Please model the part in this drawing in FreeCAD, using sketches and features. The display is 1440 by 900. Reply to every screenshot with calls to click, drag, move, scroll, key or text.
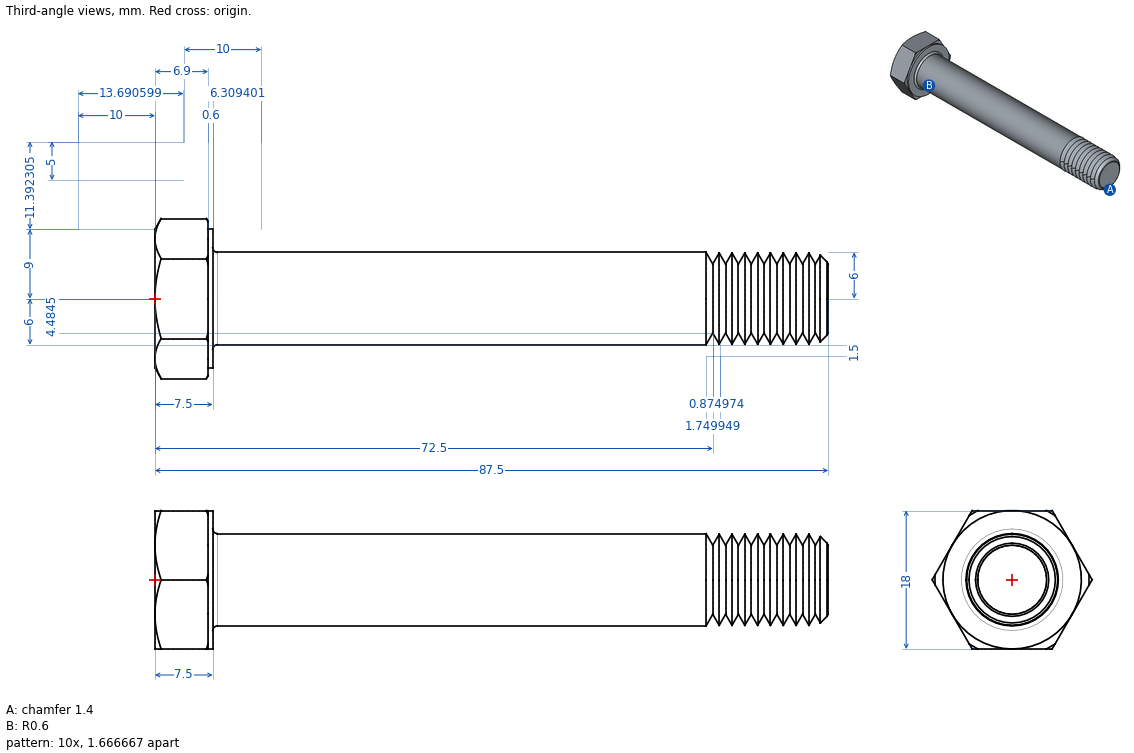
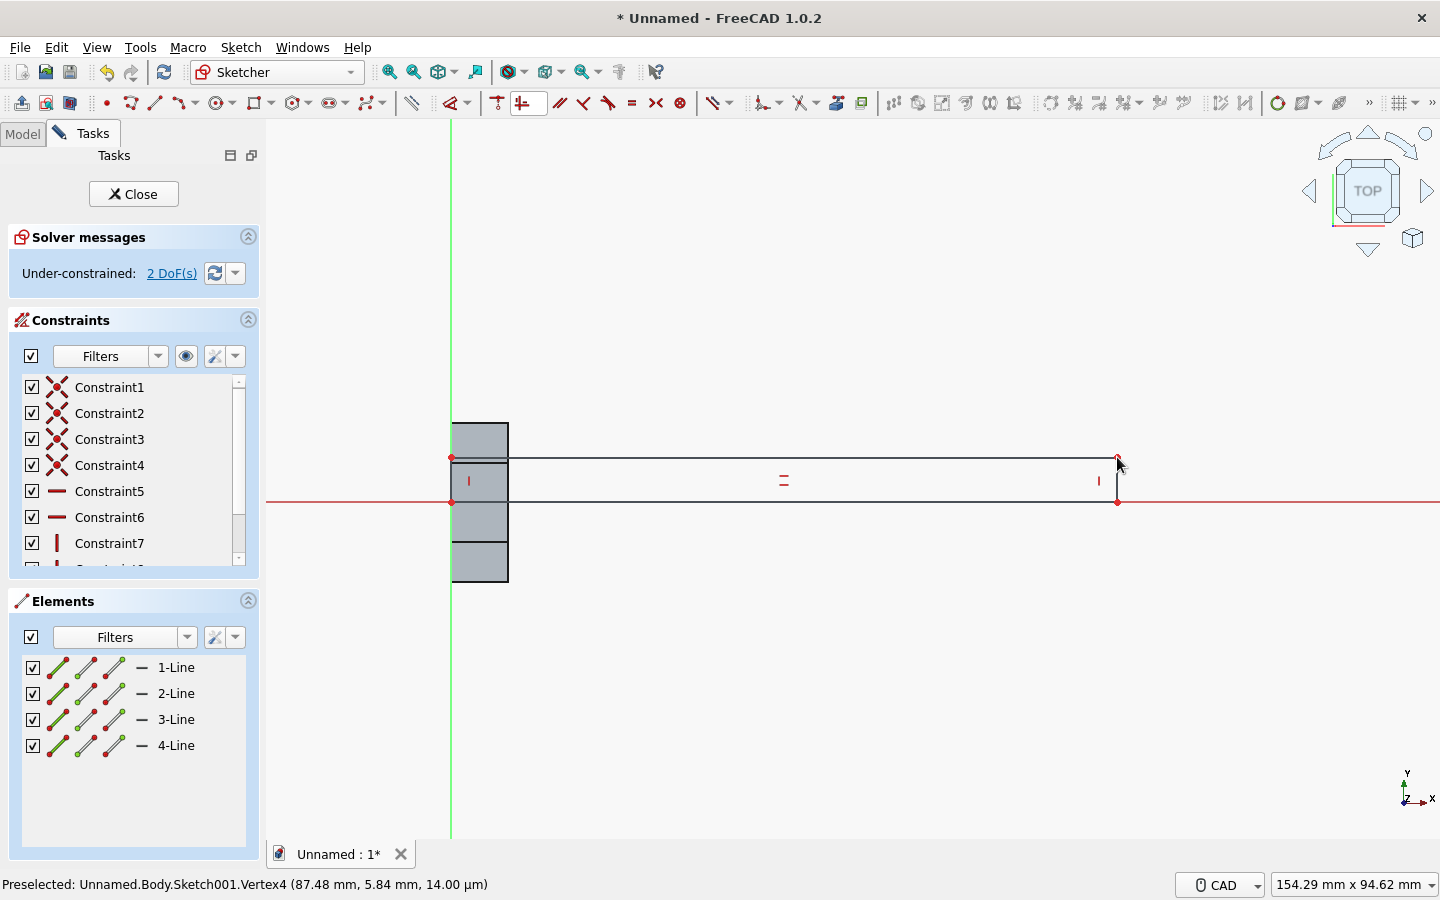
click(450, 104)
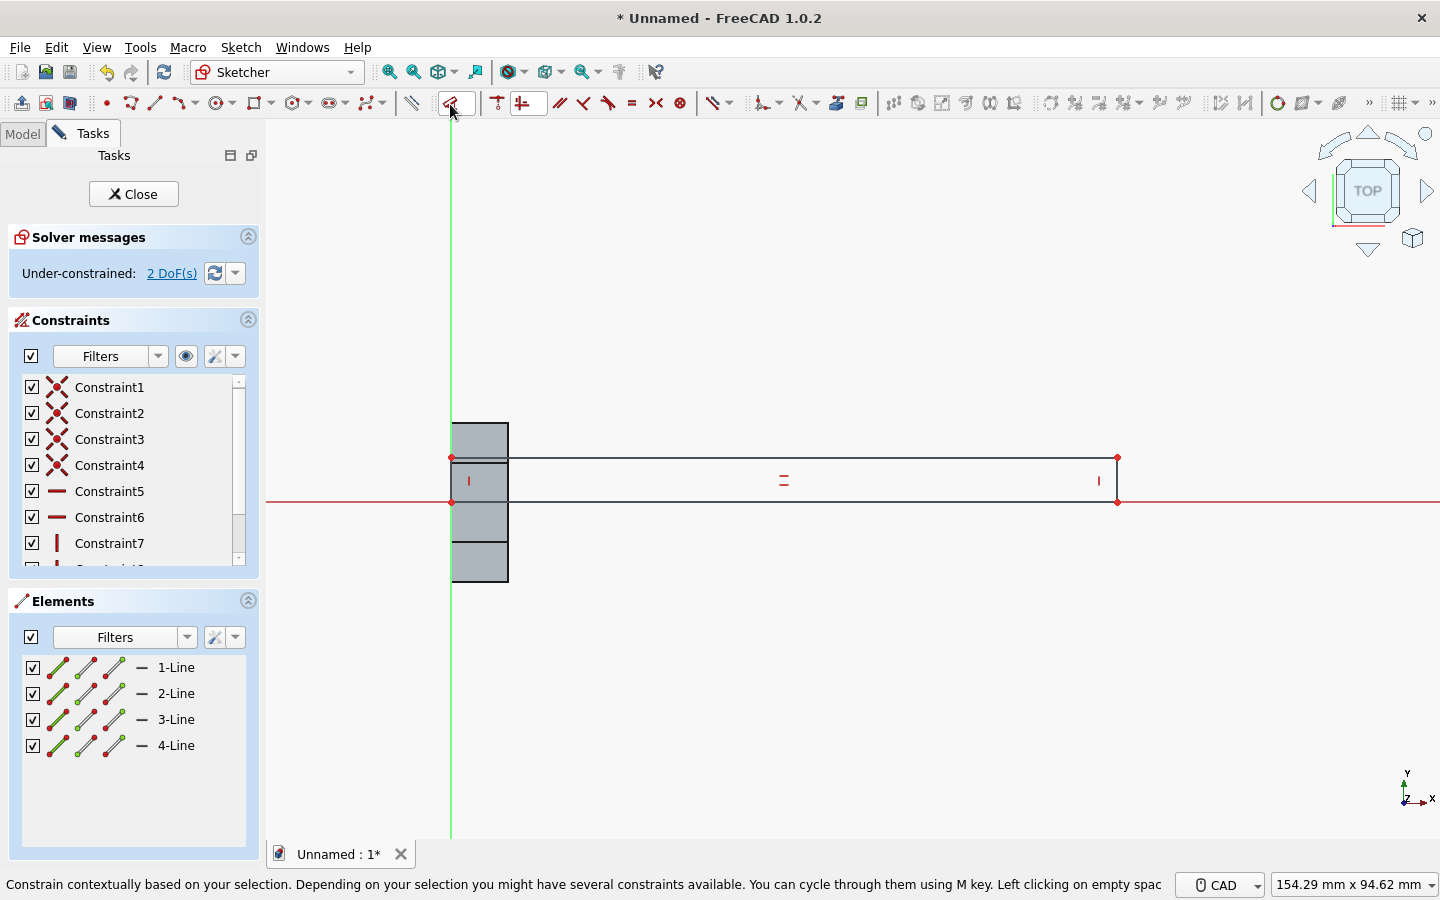
click(1117, 489)
click(1151, 480)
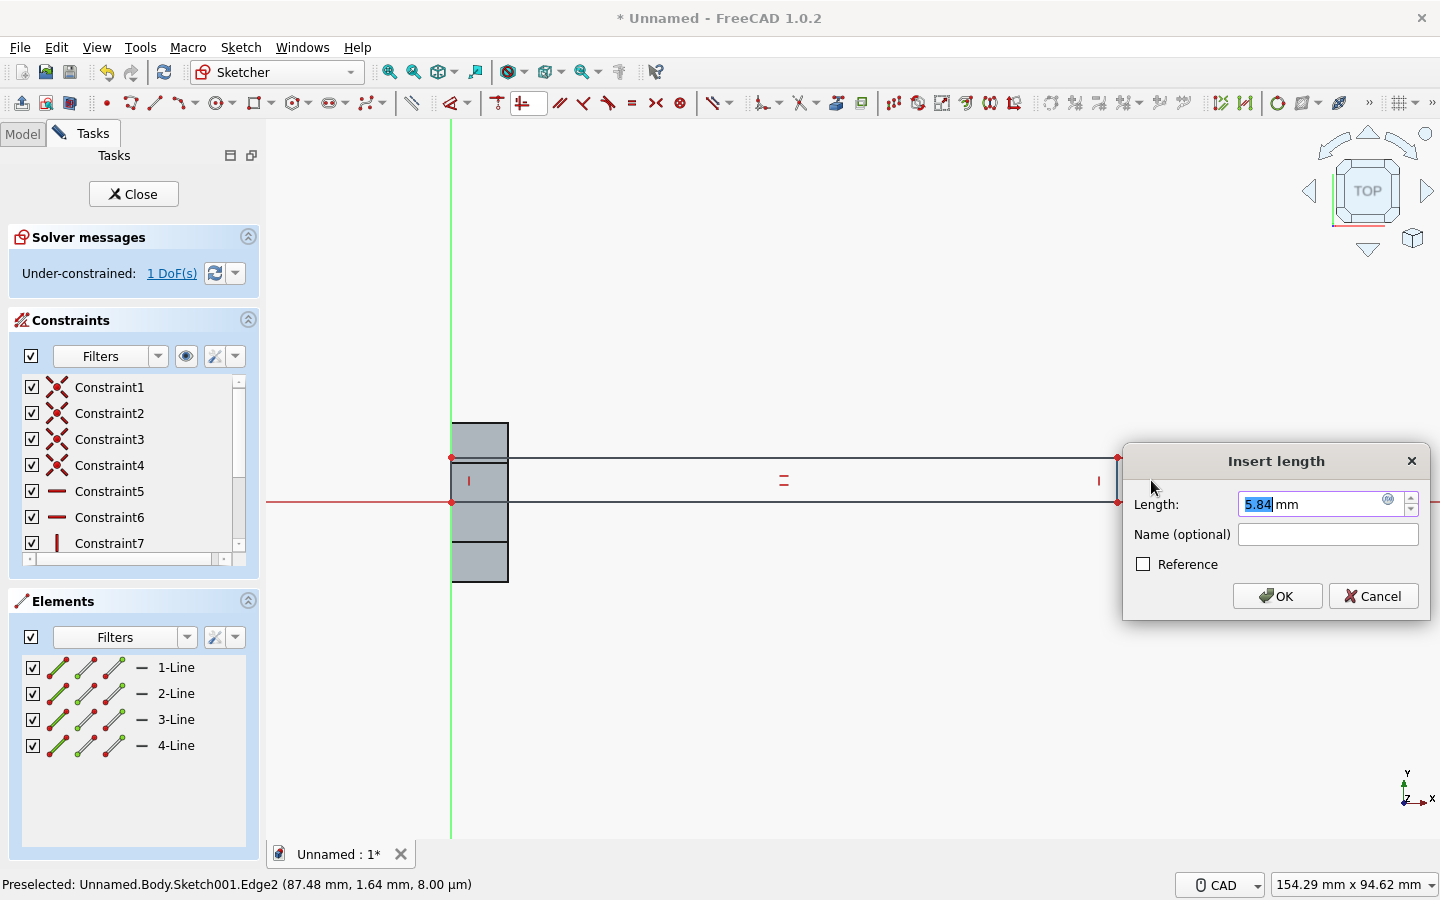
text(6)
key(Return)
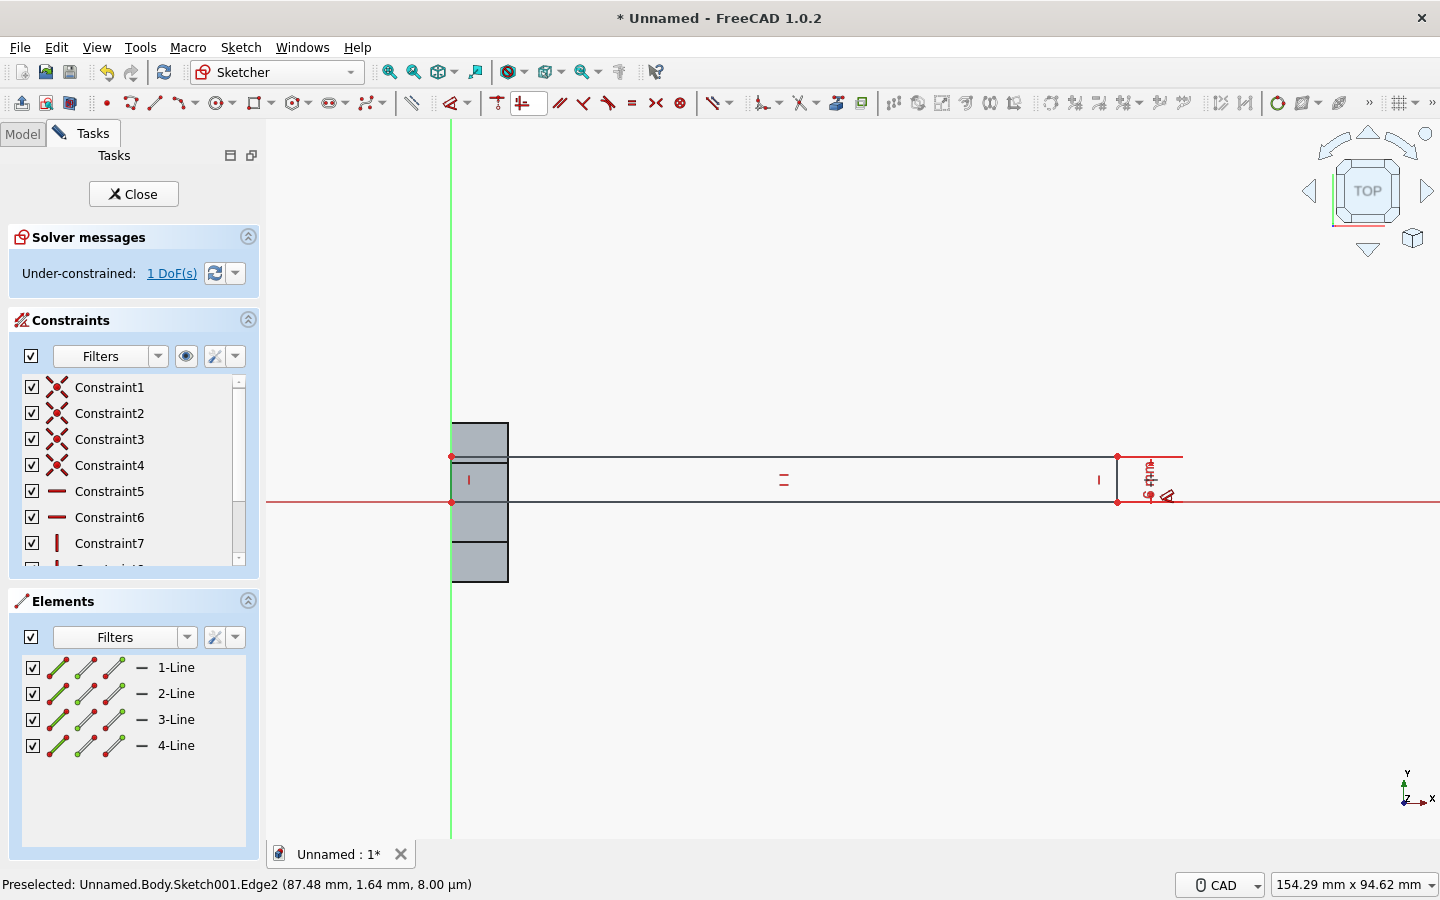
click(651, 502)
click(784, 536)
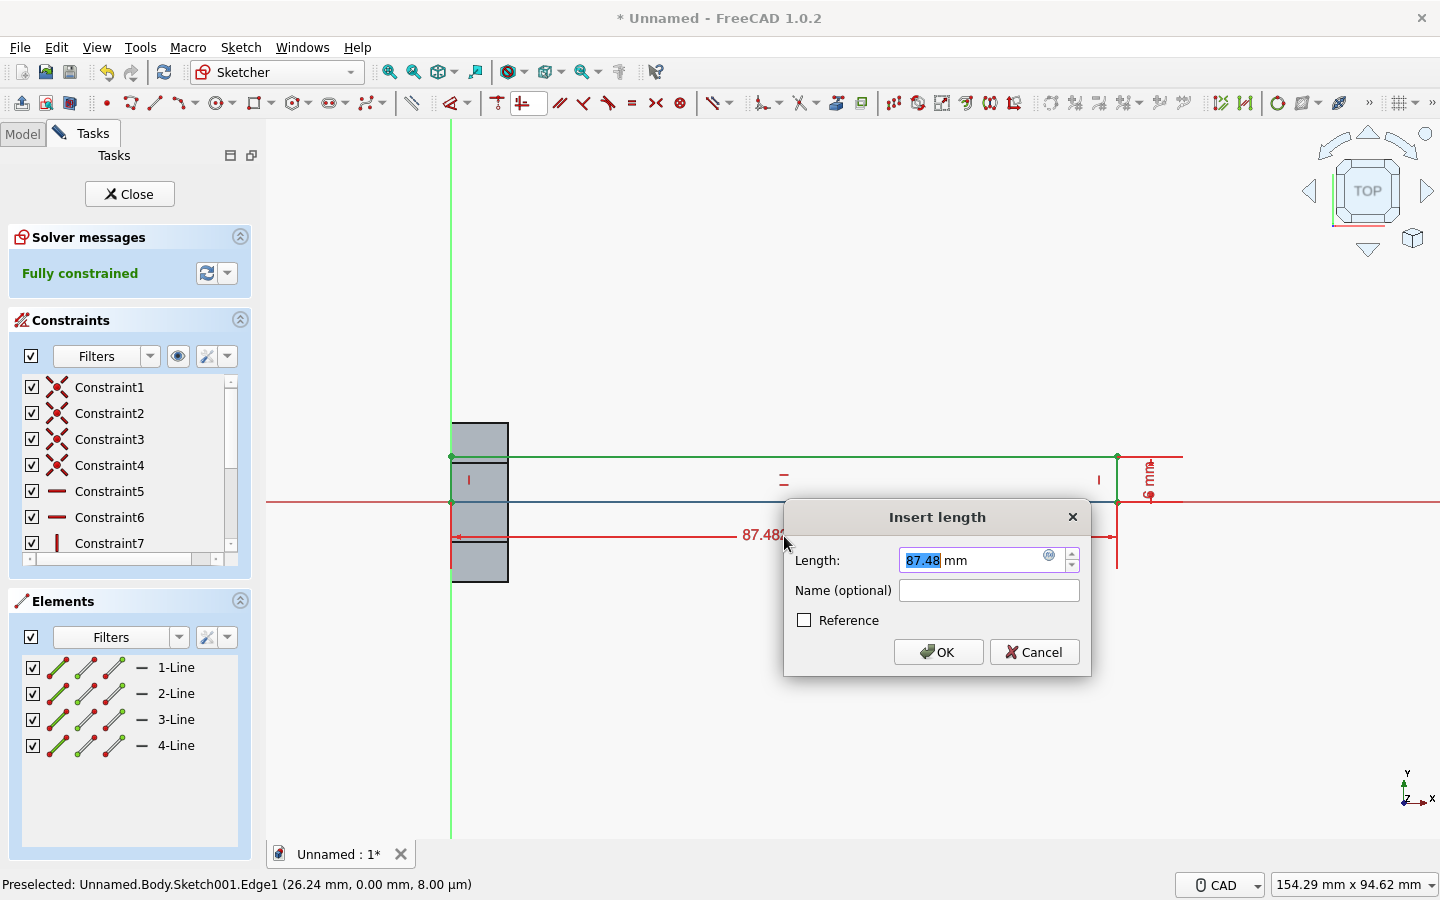
text(87.5)
key(Return)
key(Escape)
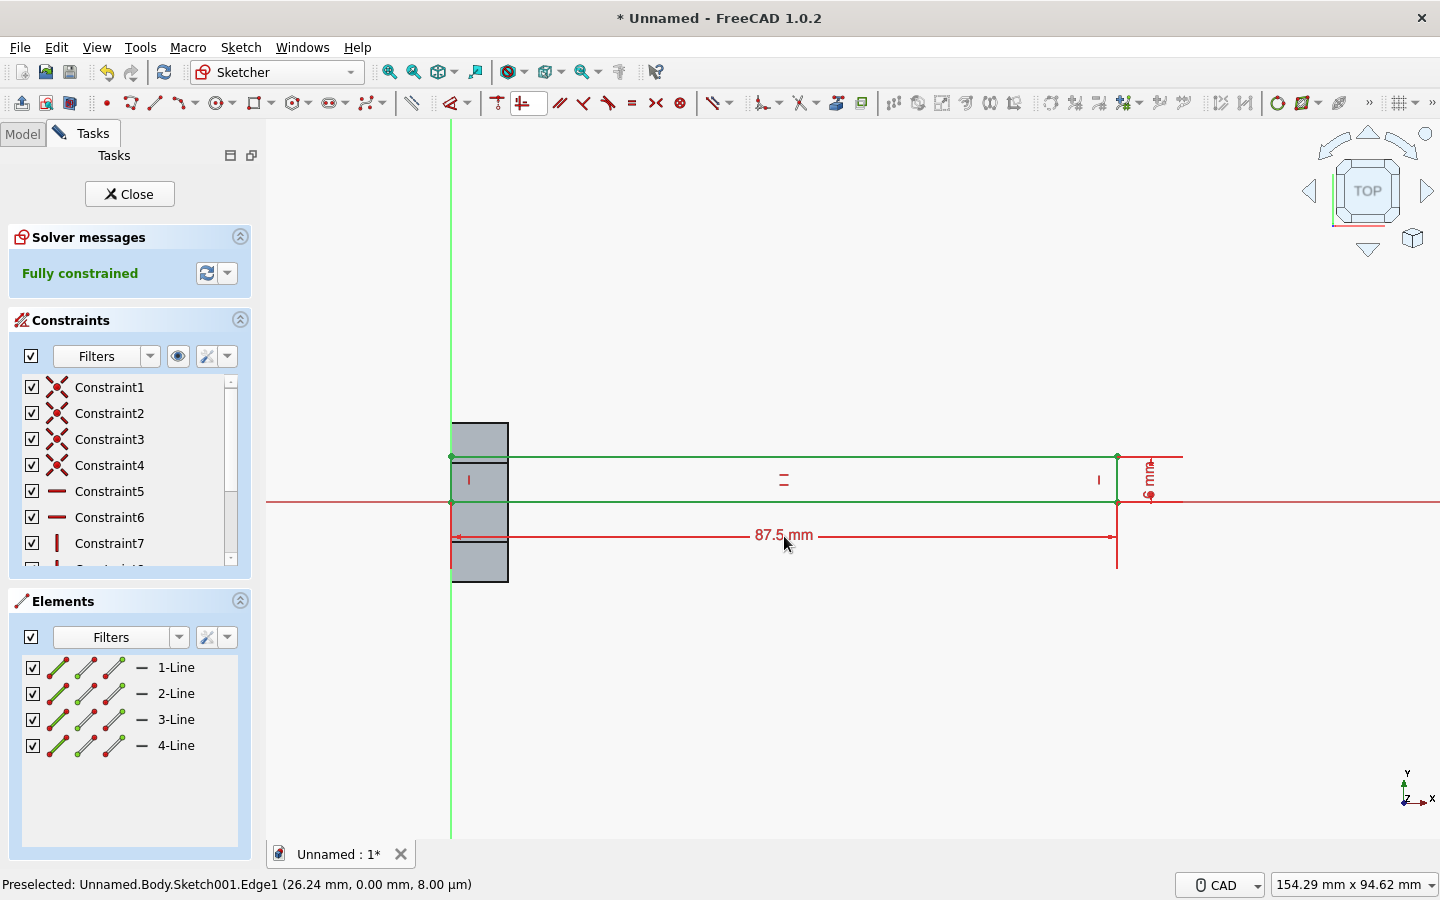
click(130, 194)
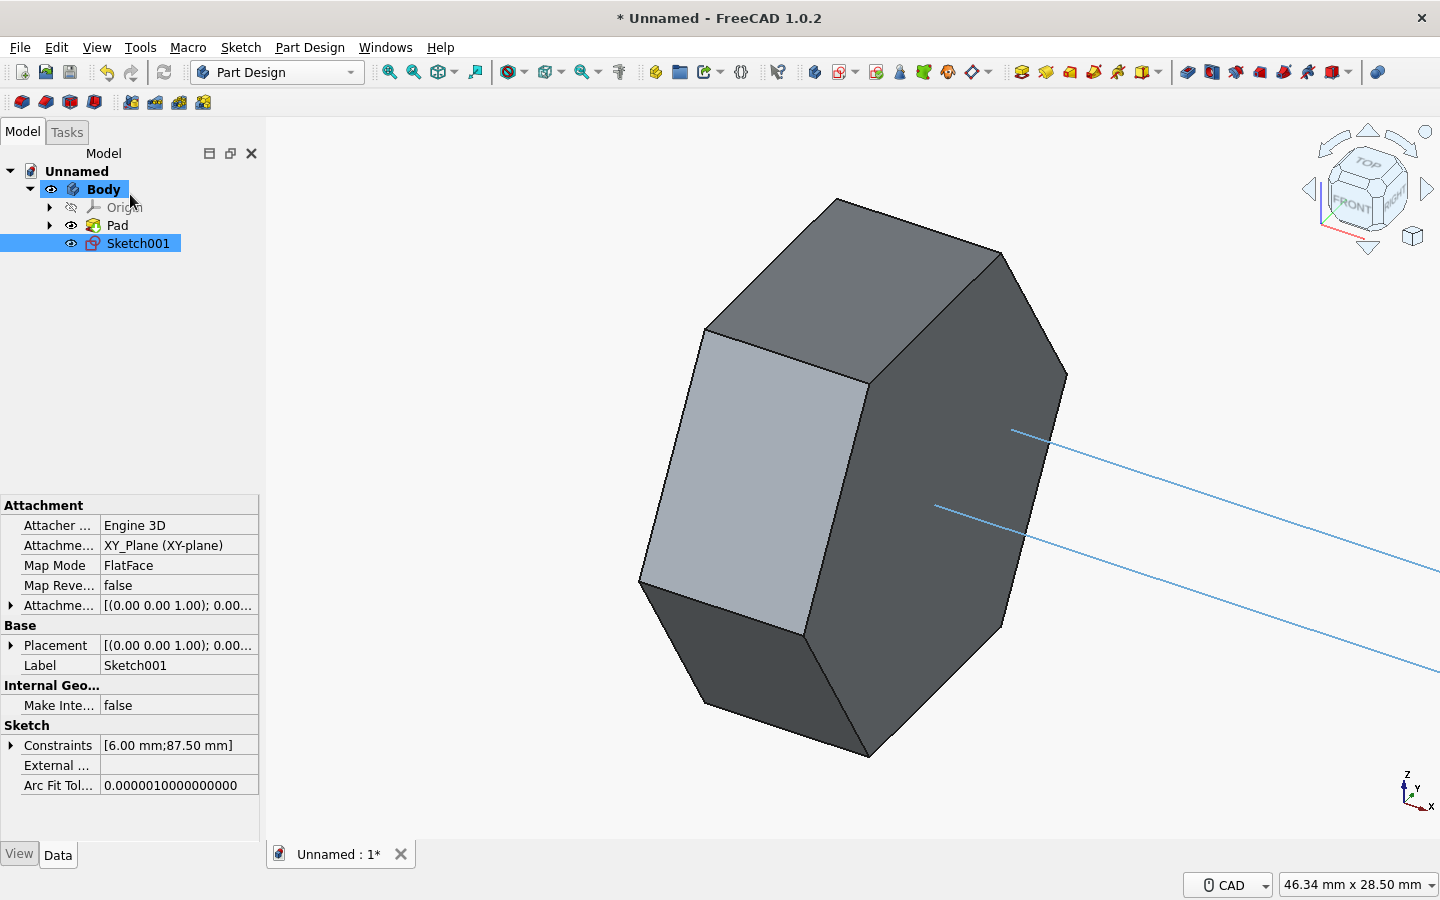
click(1046, 72)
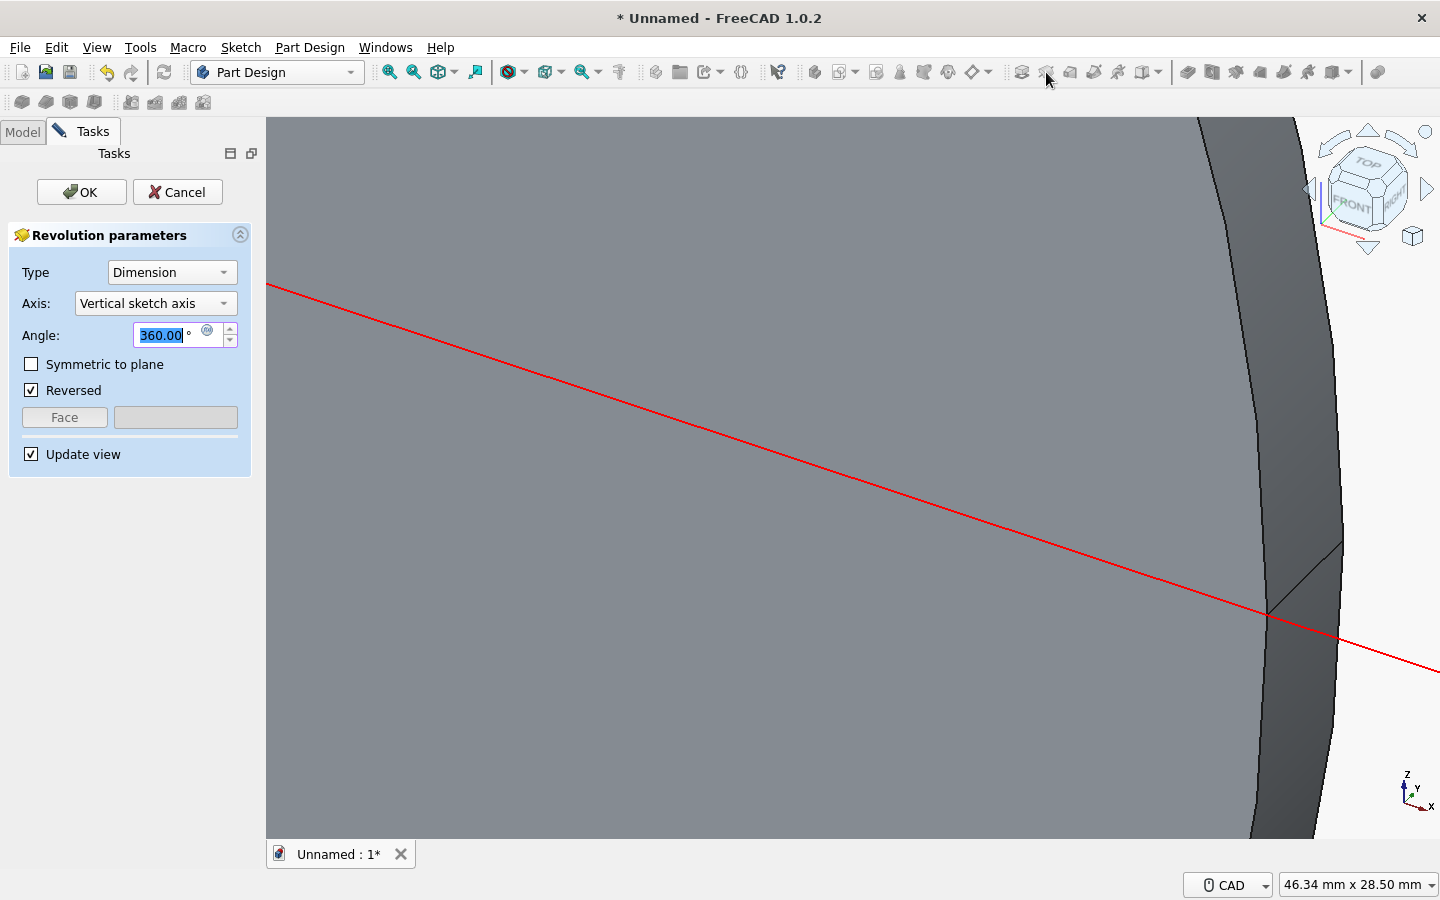
click(156, 304)